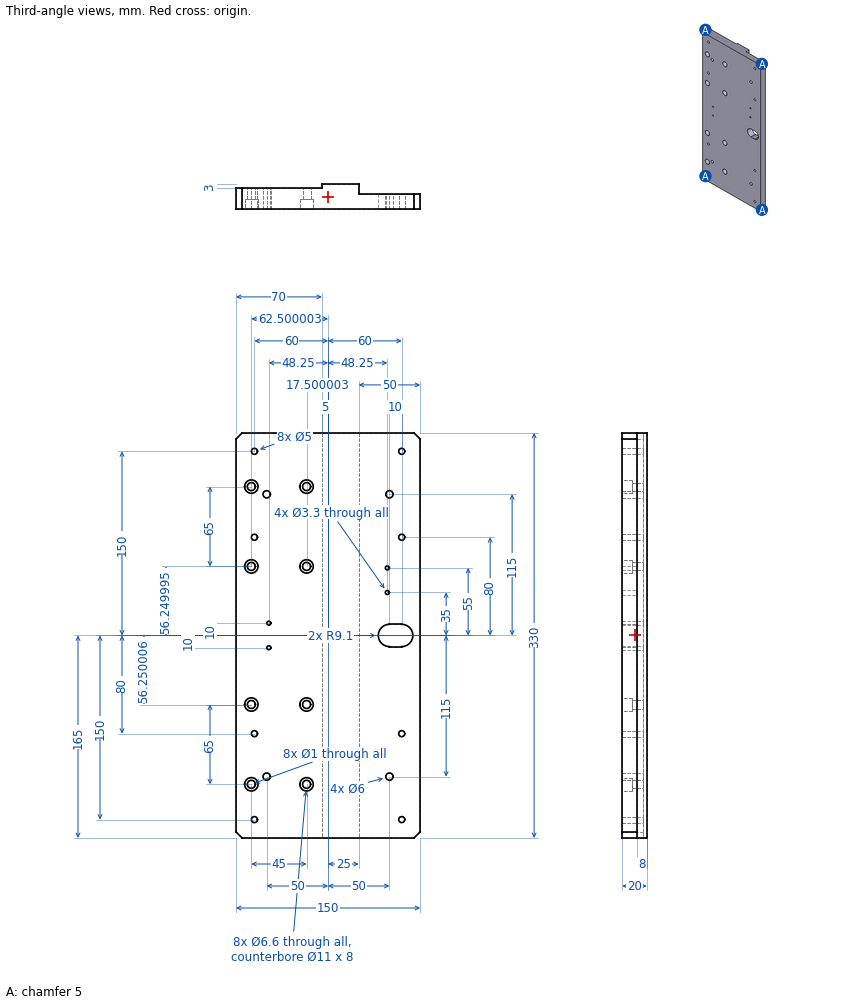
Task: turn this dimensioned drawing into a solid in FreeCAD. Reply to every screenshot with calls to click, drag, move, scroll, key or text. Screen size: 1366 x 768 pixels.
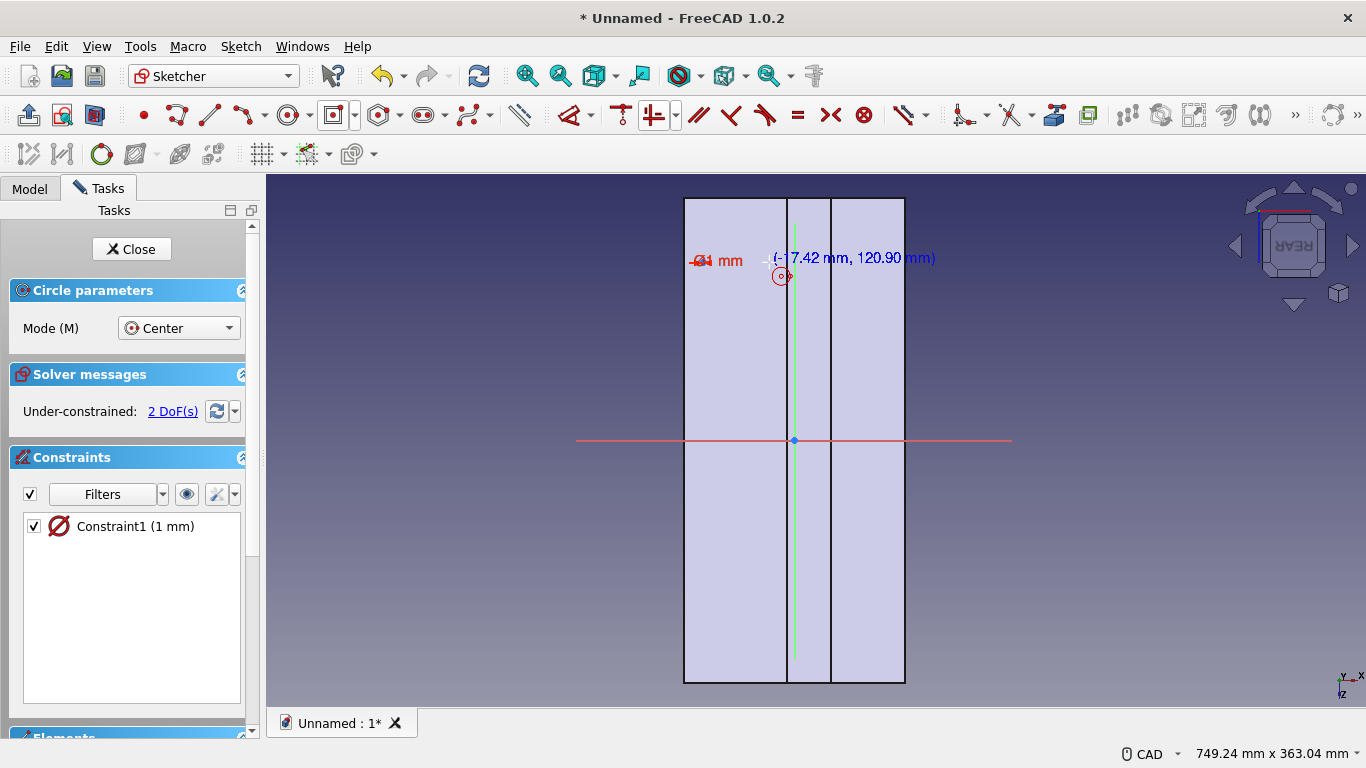
click(769, 262)
move(769, 262)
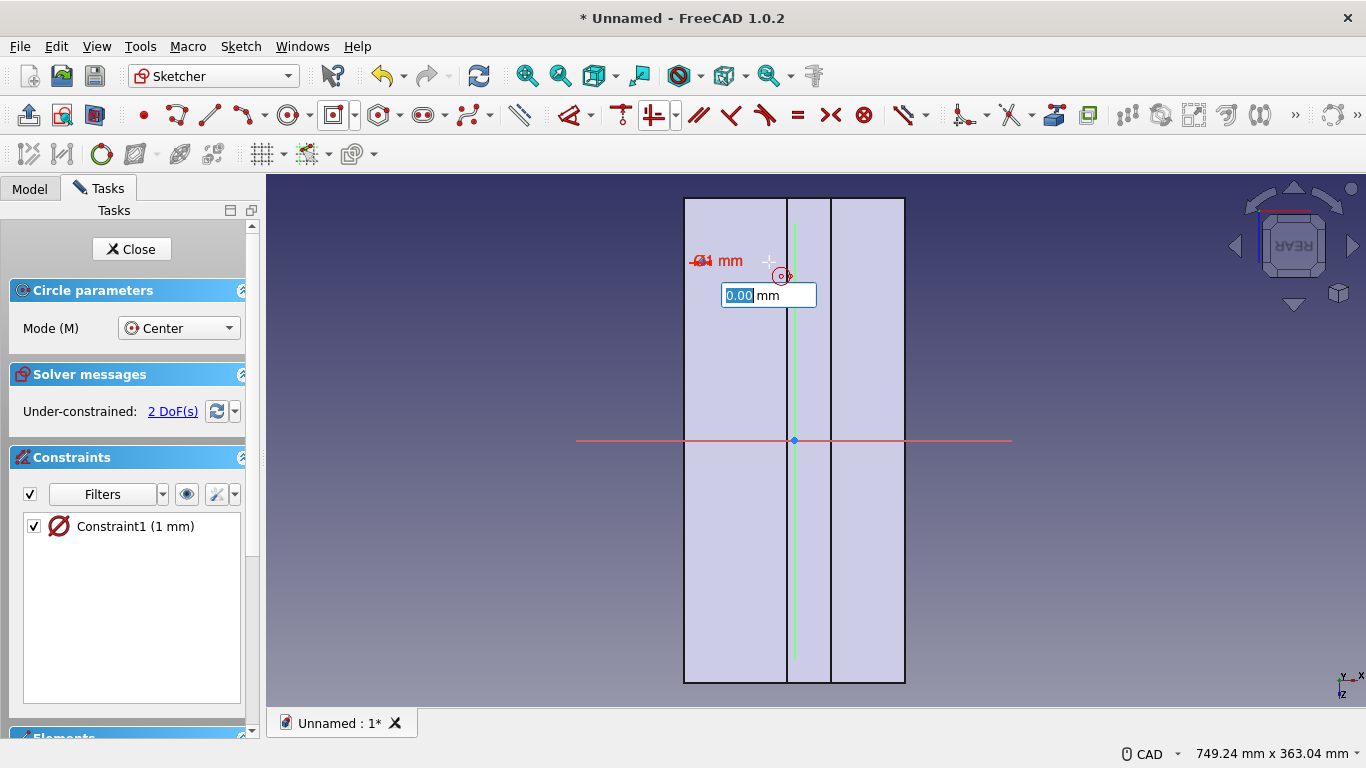
text(1)
key(Return)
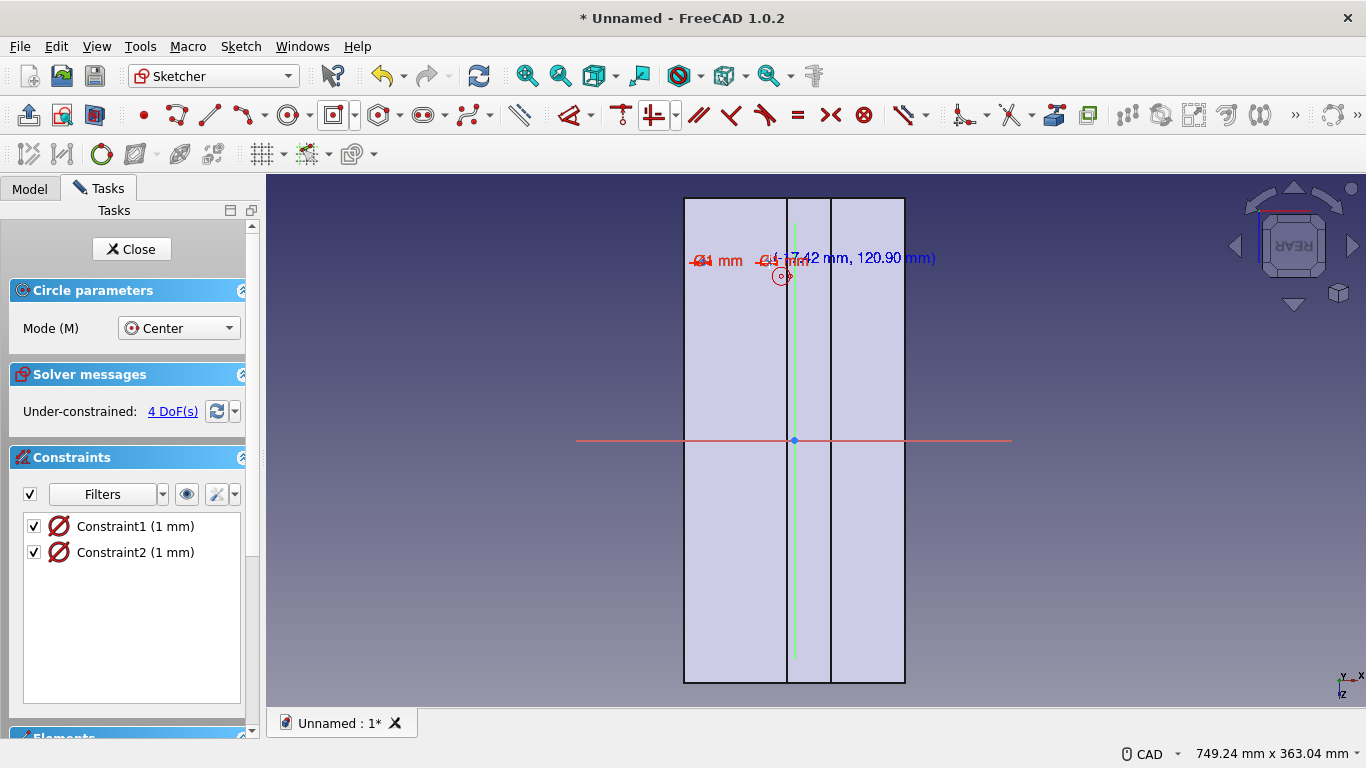
scroll(703, 358, up, 18)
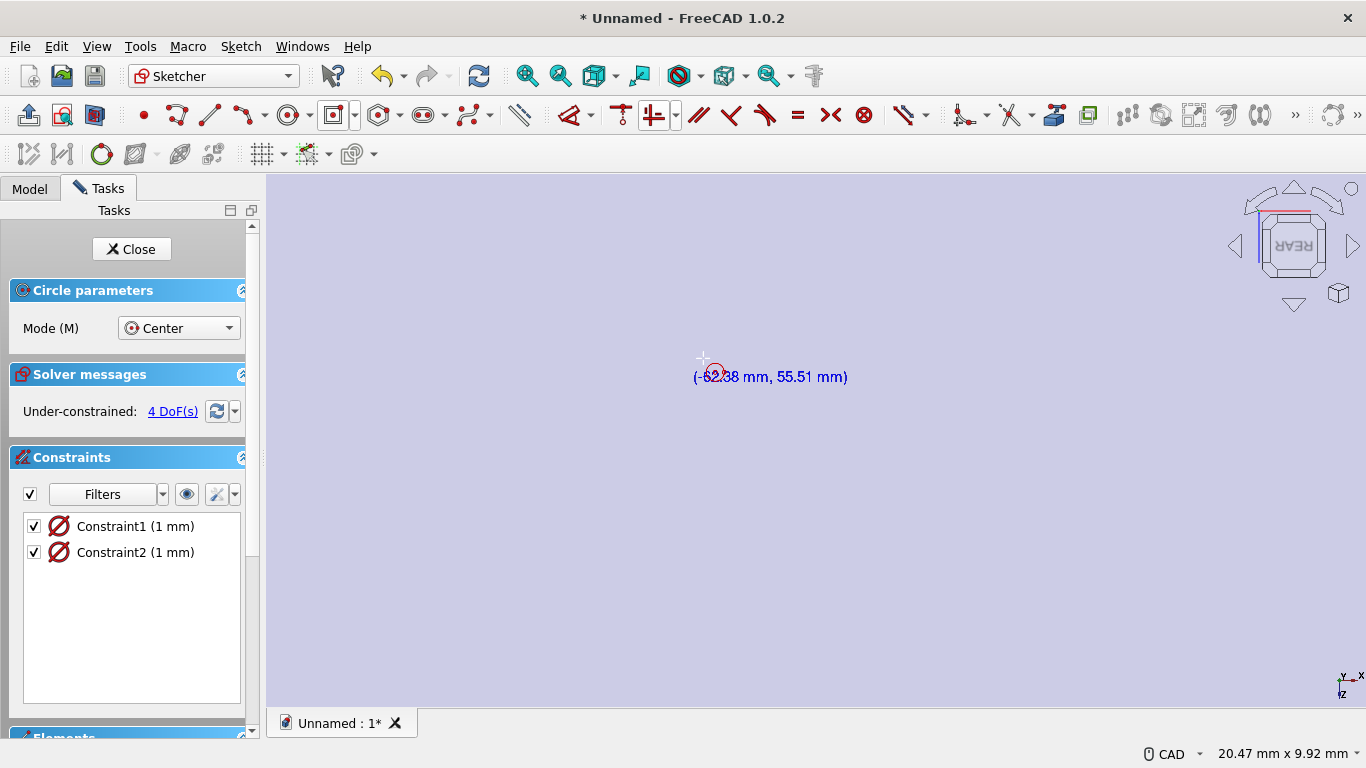
scroll(703, 358, down, 18)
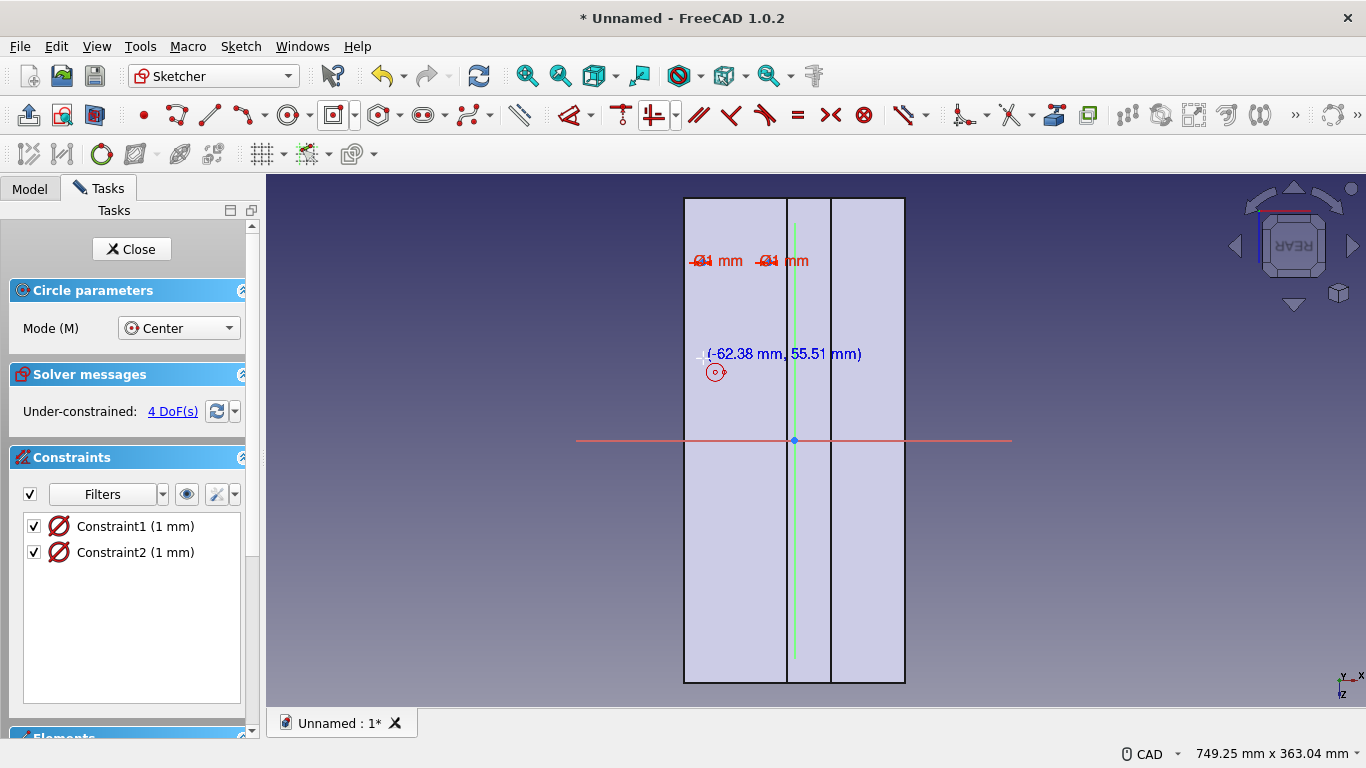
click(703, 358)
move(703, 357)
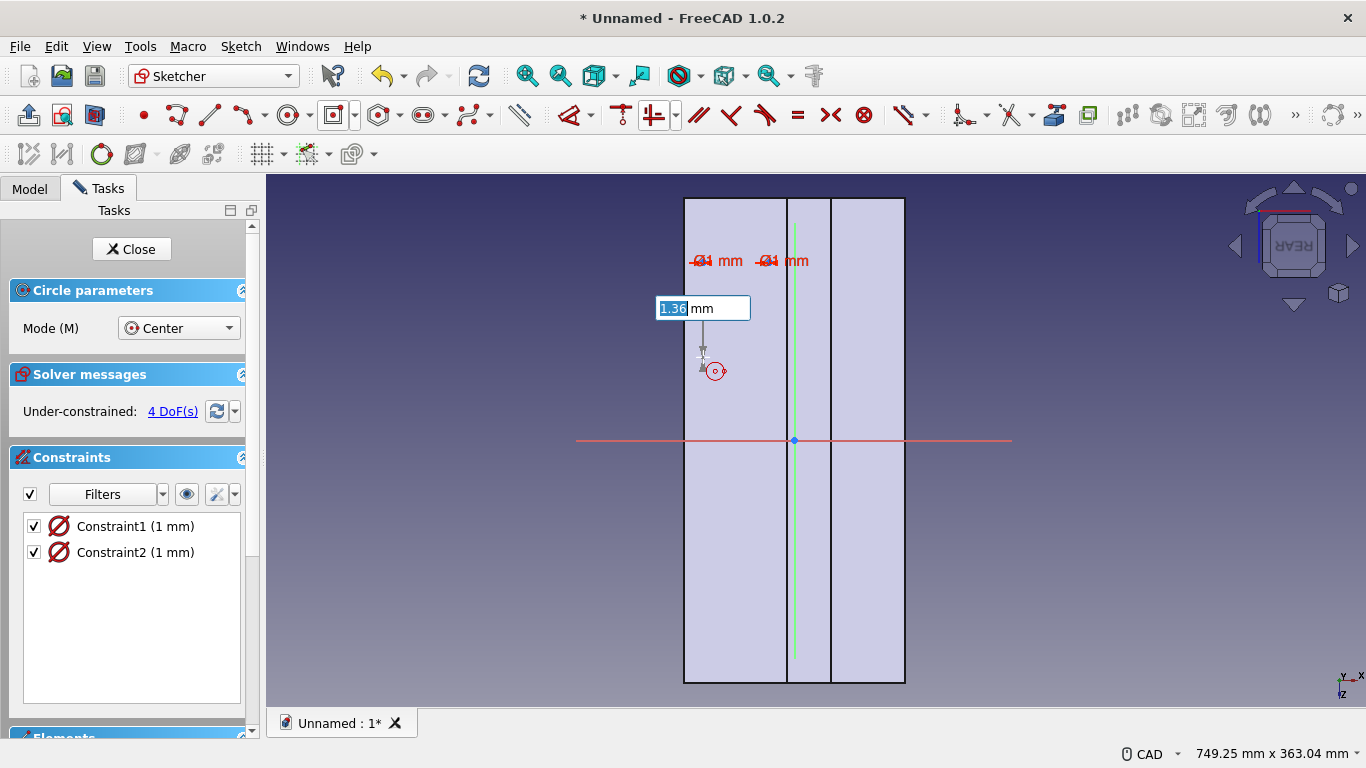
text(1)
key(Return)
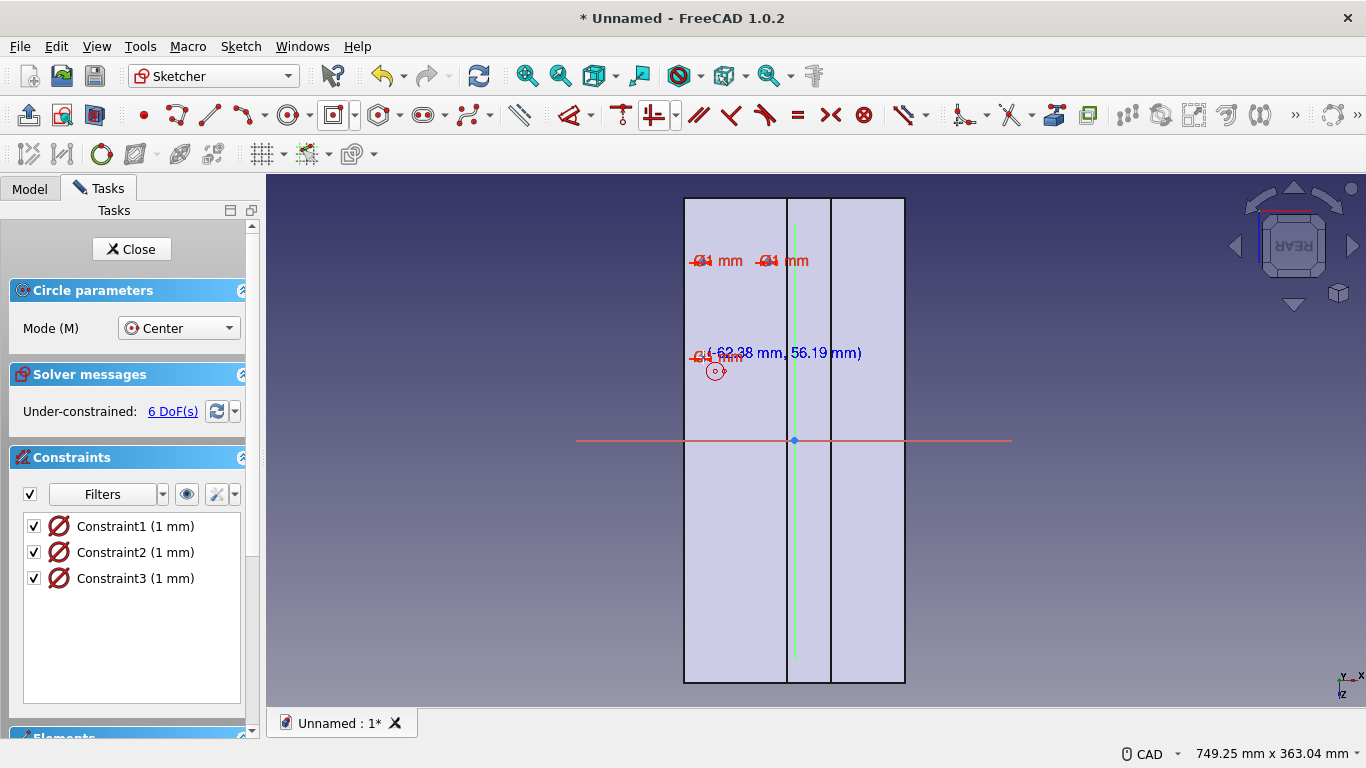
scroll(769, 358, up, 18)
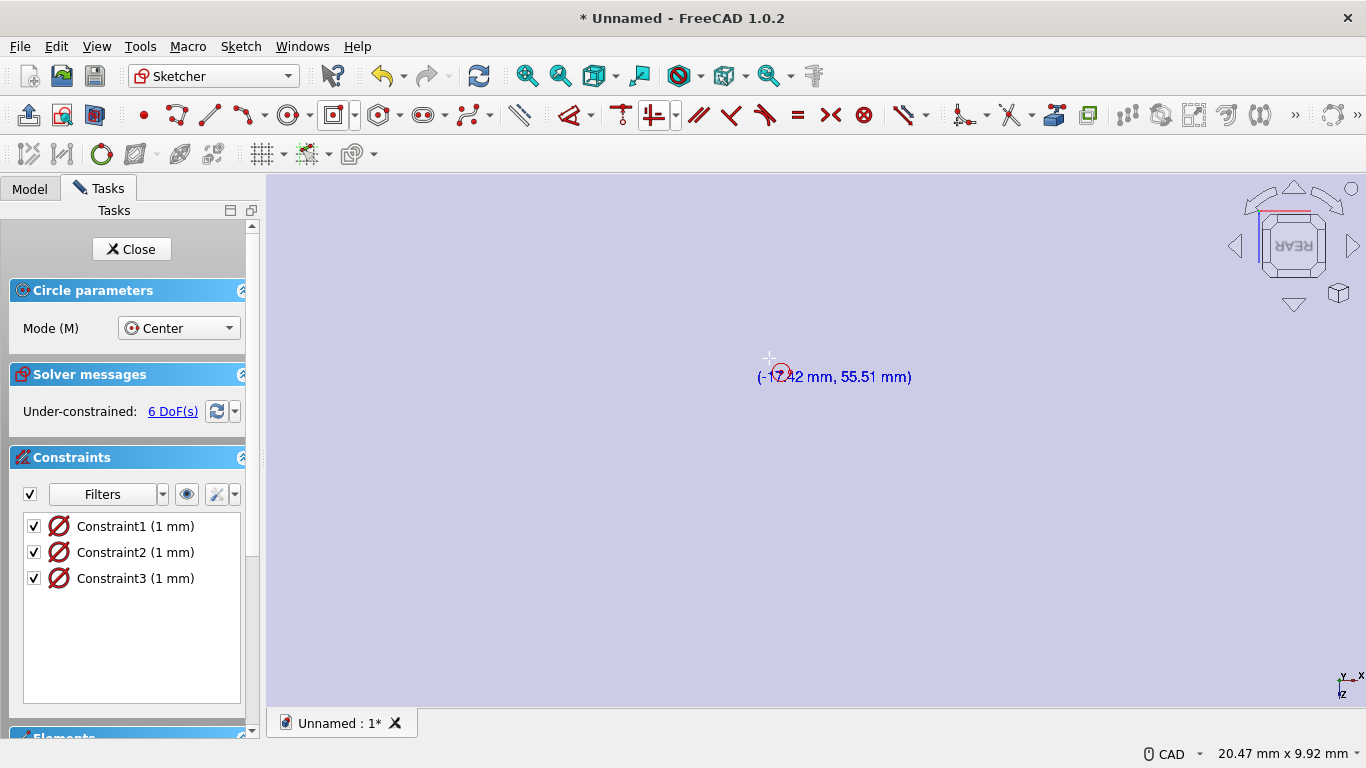
scroll(769, 358, down, 18)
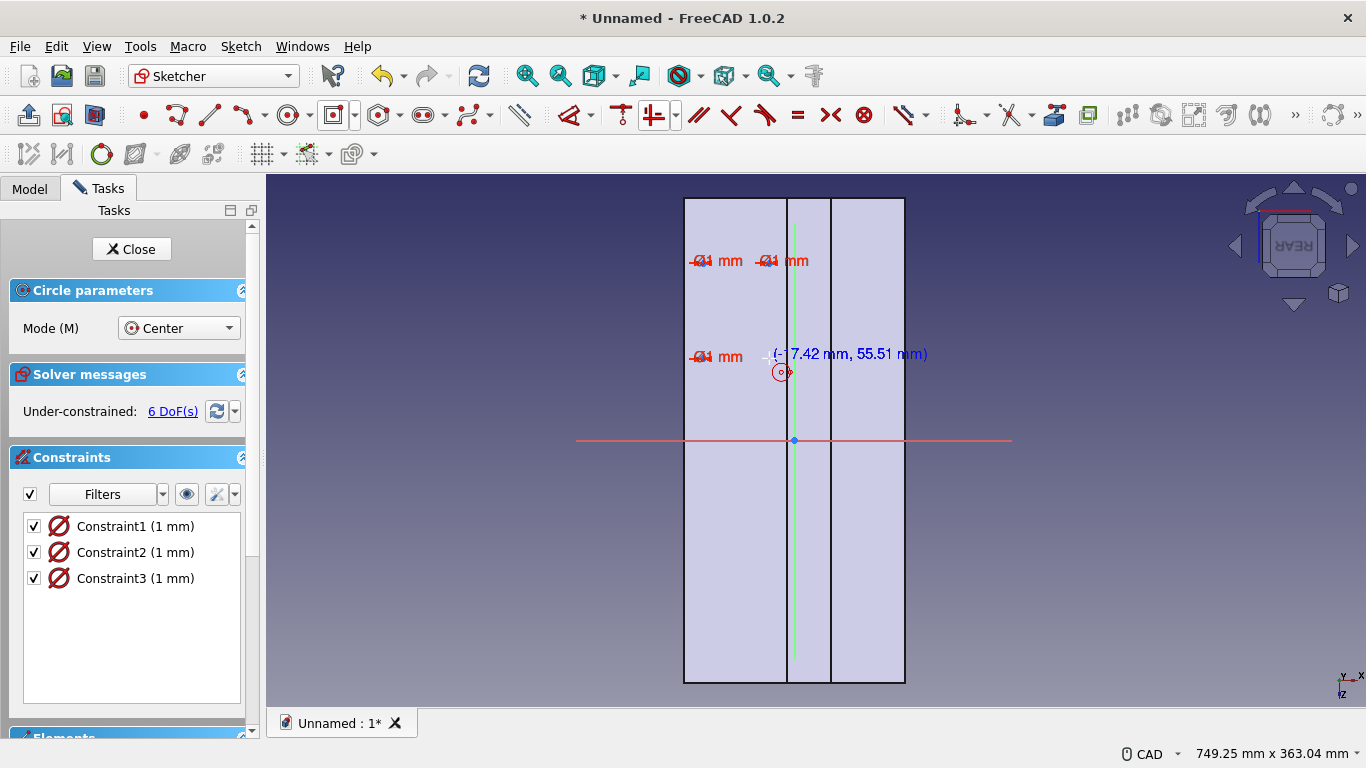
click(769, 358)
move(769, 357)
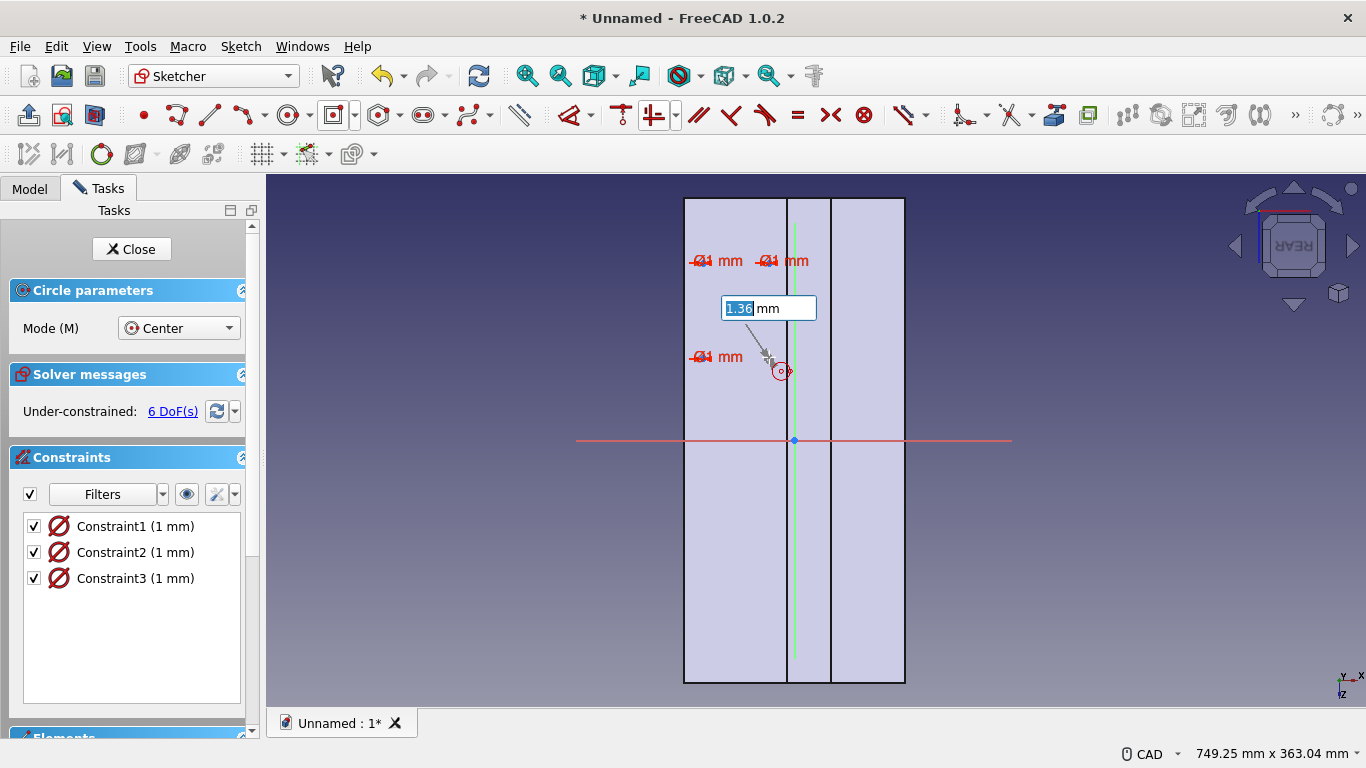
text(1)
key(Return)